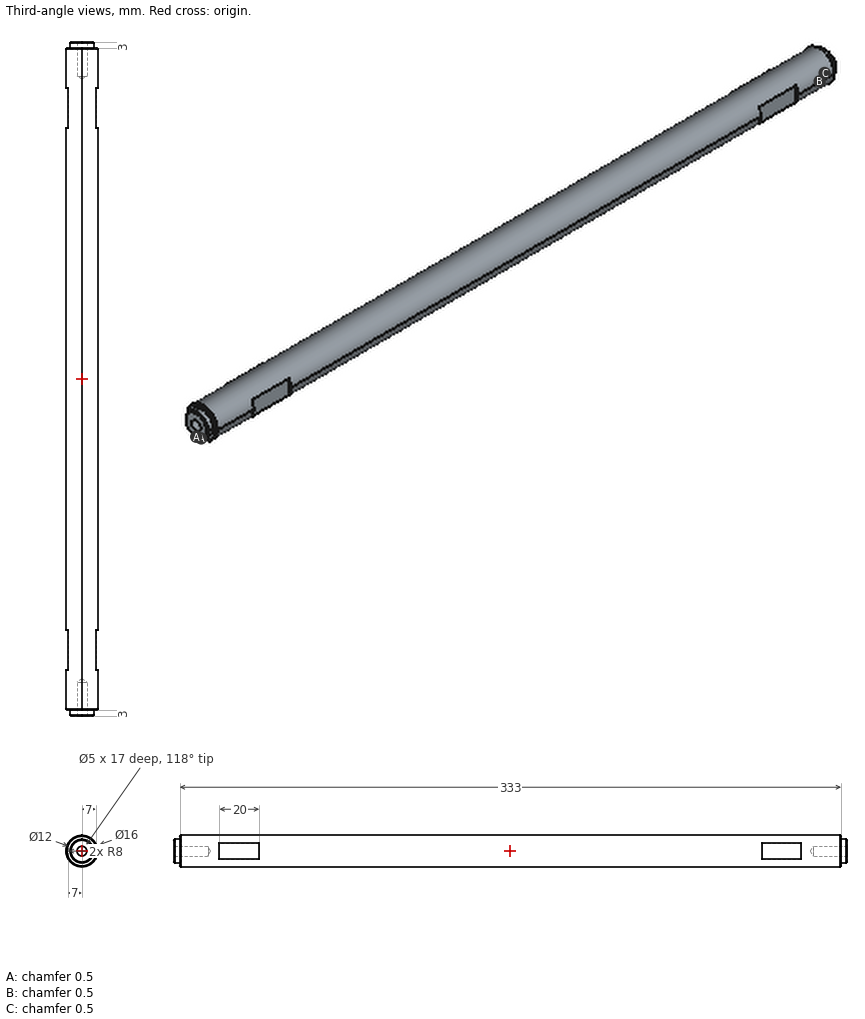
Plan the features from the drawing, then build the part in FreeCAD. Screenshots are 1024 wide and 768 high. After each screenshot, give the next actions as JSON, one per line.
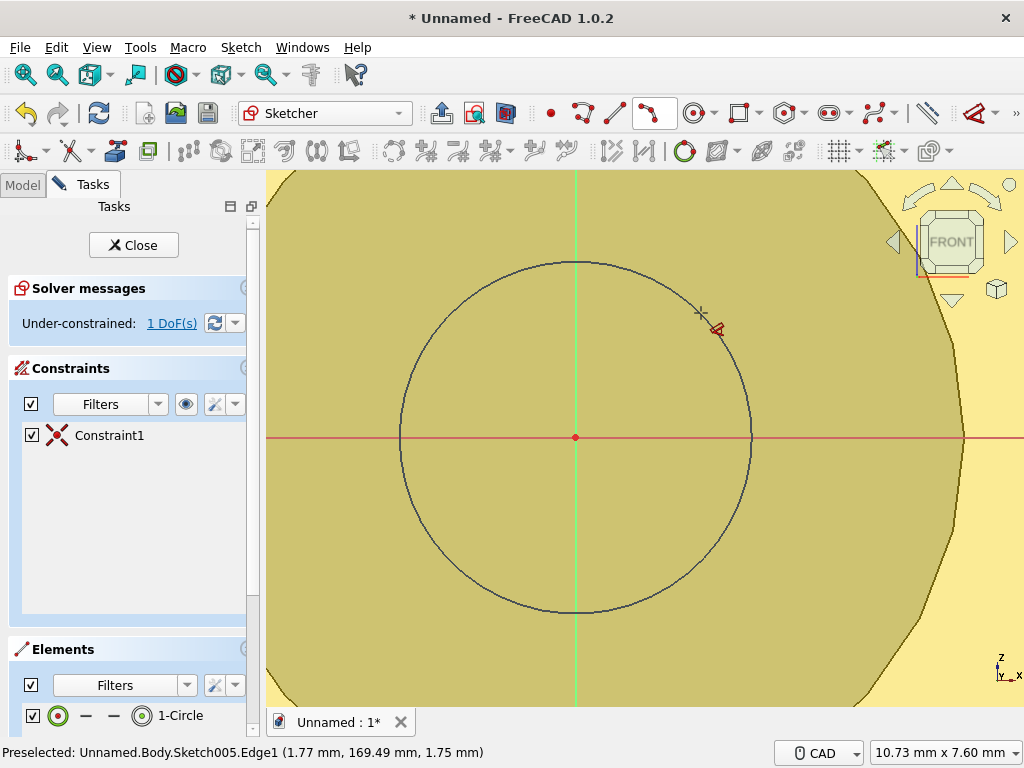
{"action": "left_click", "coordinate": [700, 313]}
{"action": "left_click", "coordinate": [723, 290]}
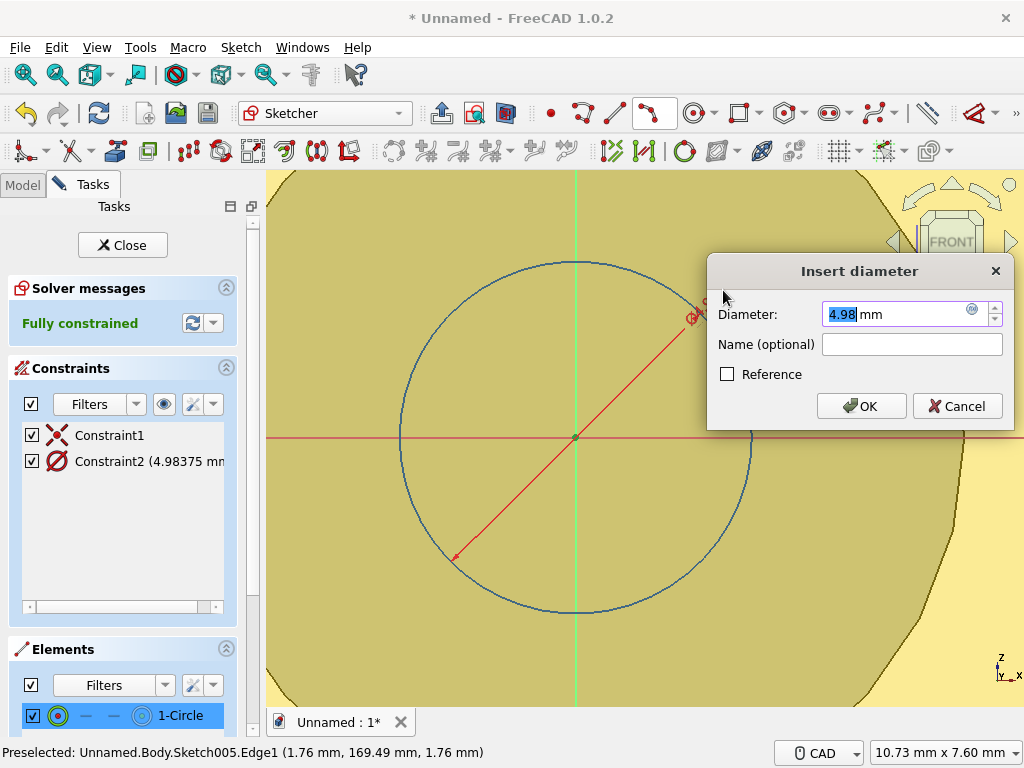
{"action": "type", "text": "5"}
{"action": "key", "text": "Return"}
{"action": "key", "text": "Escape"}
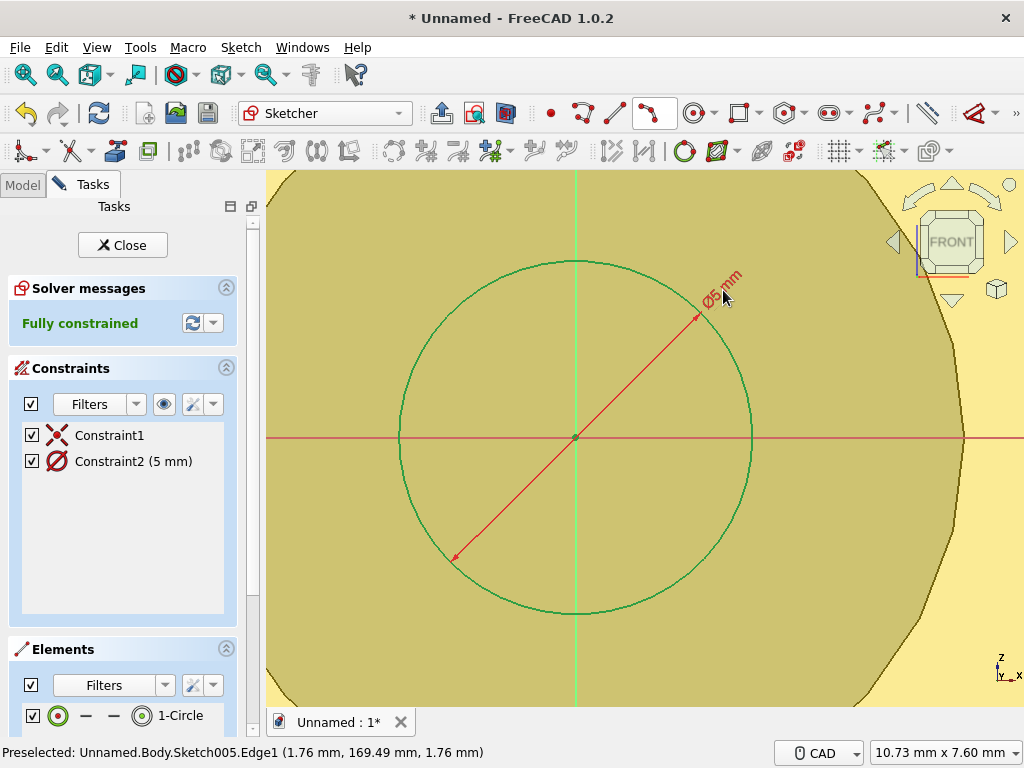
{"action": "left_click", "coordinate": [123, 245]}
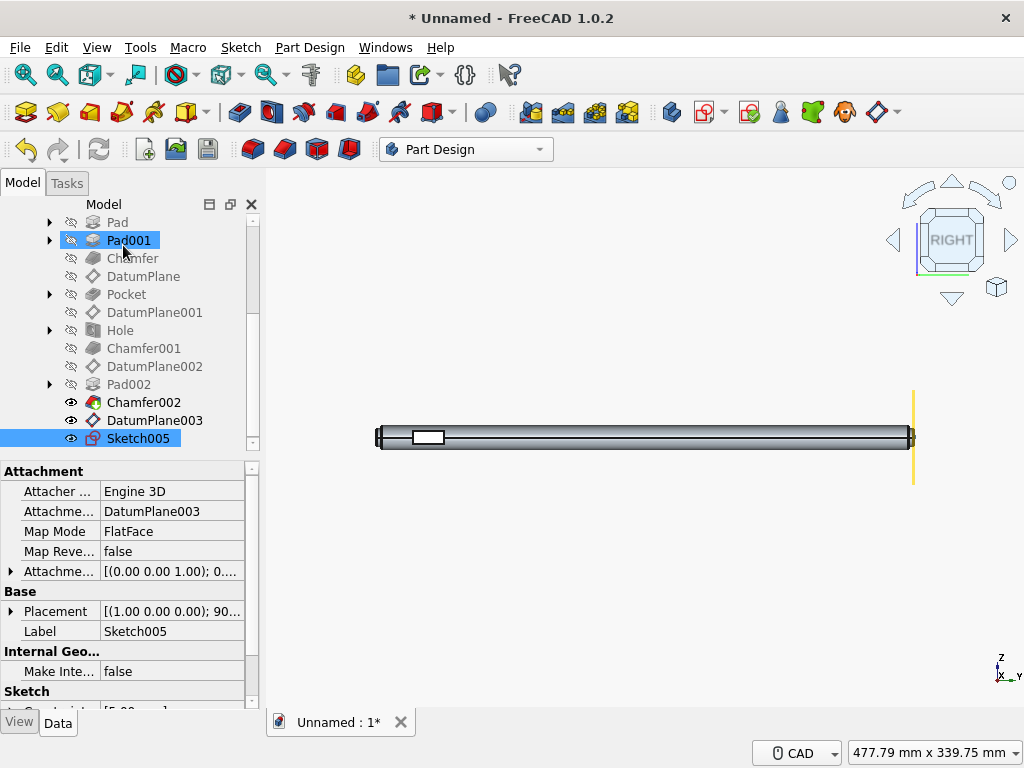
{"action": "left_click", "coordinate": [272, 112]}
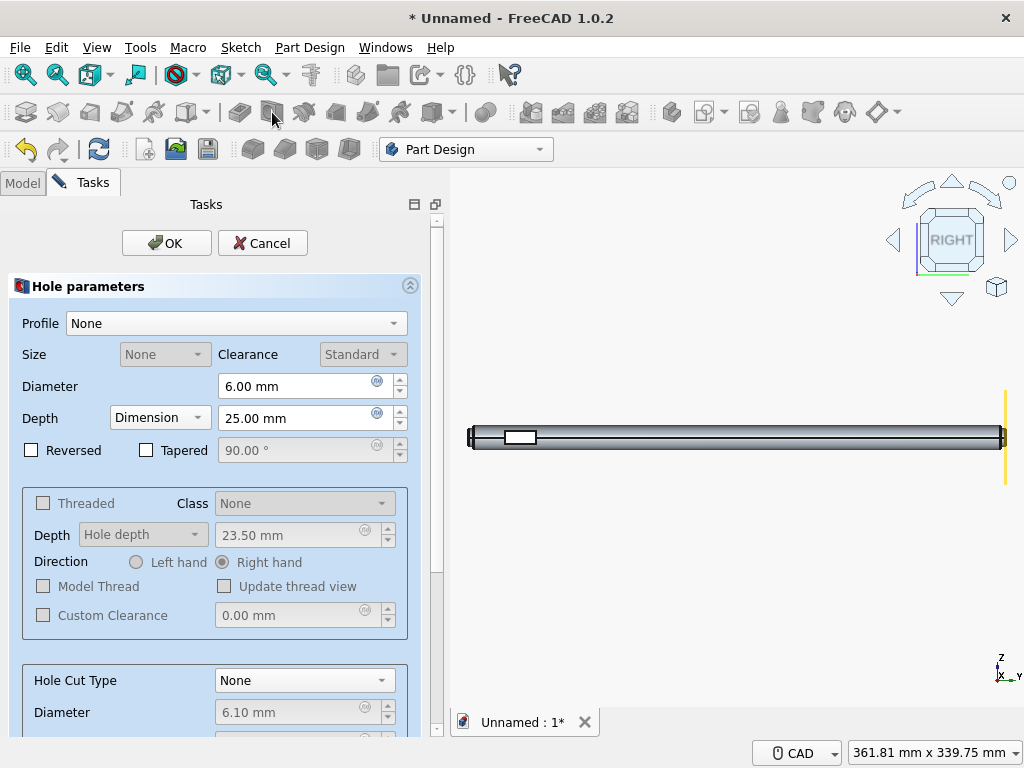
{"action": "triple_click", "coordinate": [305, 386]}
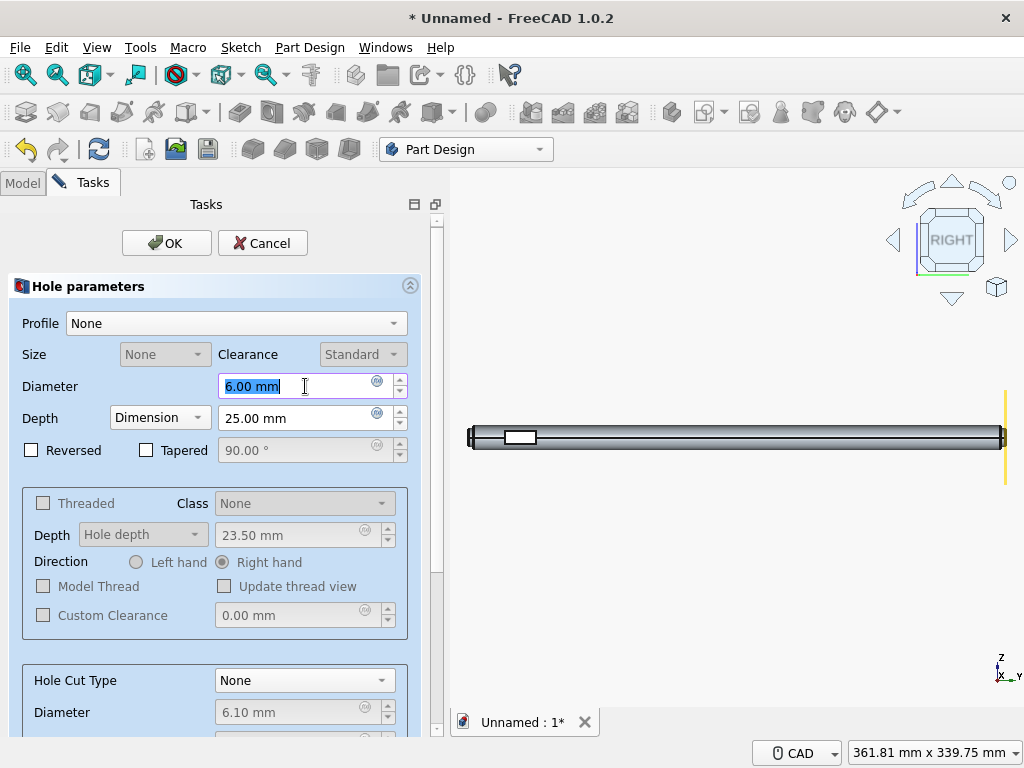
{"action": "type", "text": "5"}
{"action": "key", "text": "Tab"}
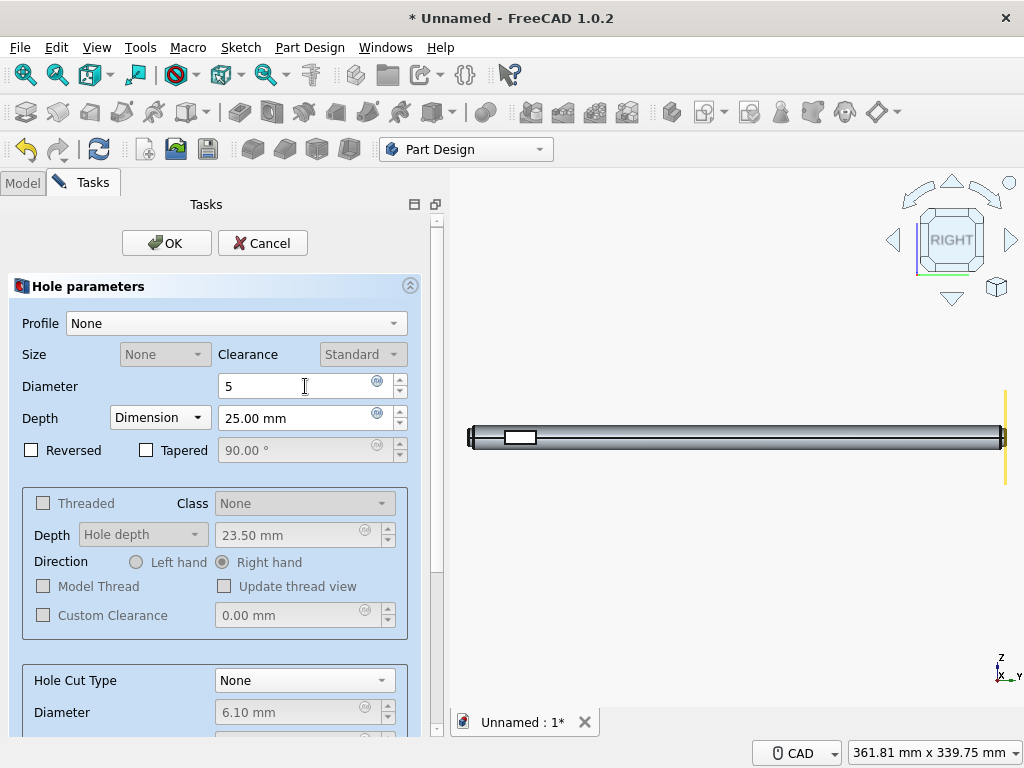
{"action": "triple_click", "coordinate": [305, 418]}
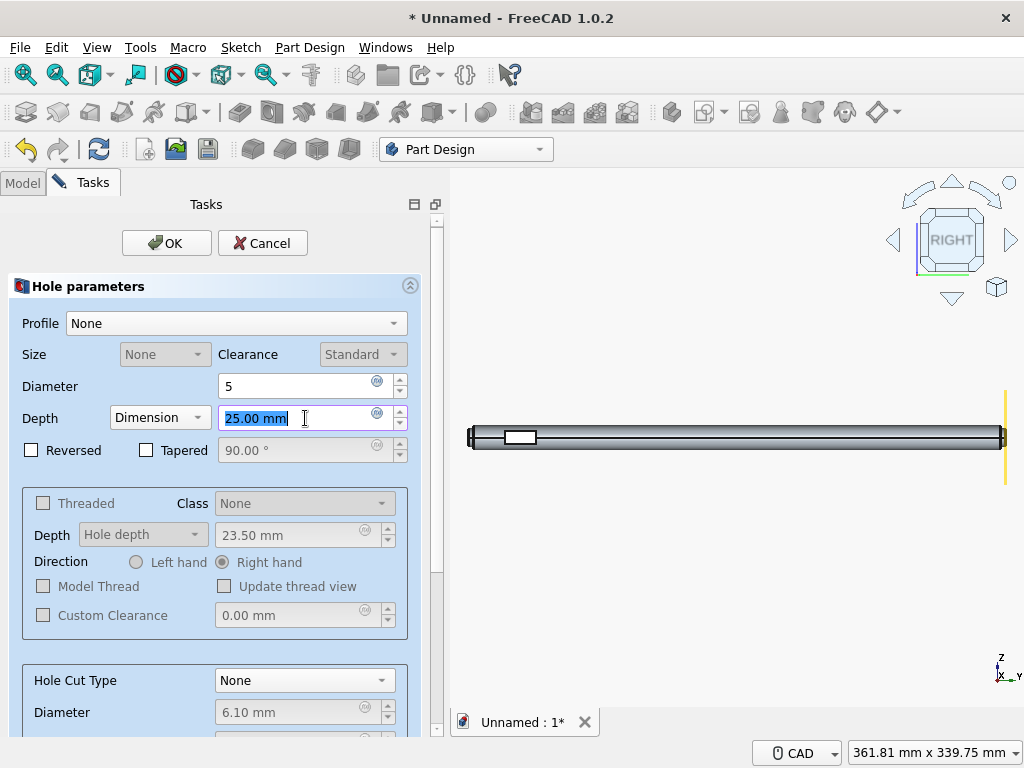
{"action": "type", "text": "17"}
{"action": "key", "text": "Tab"}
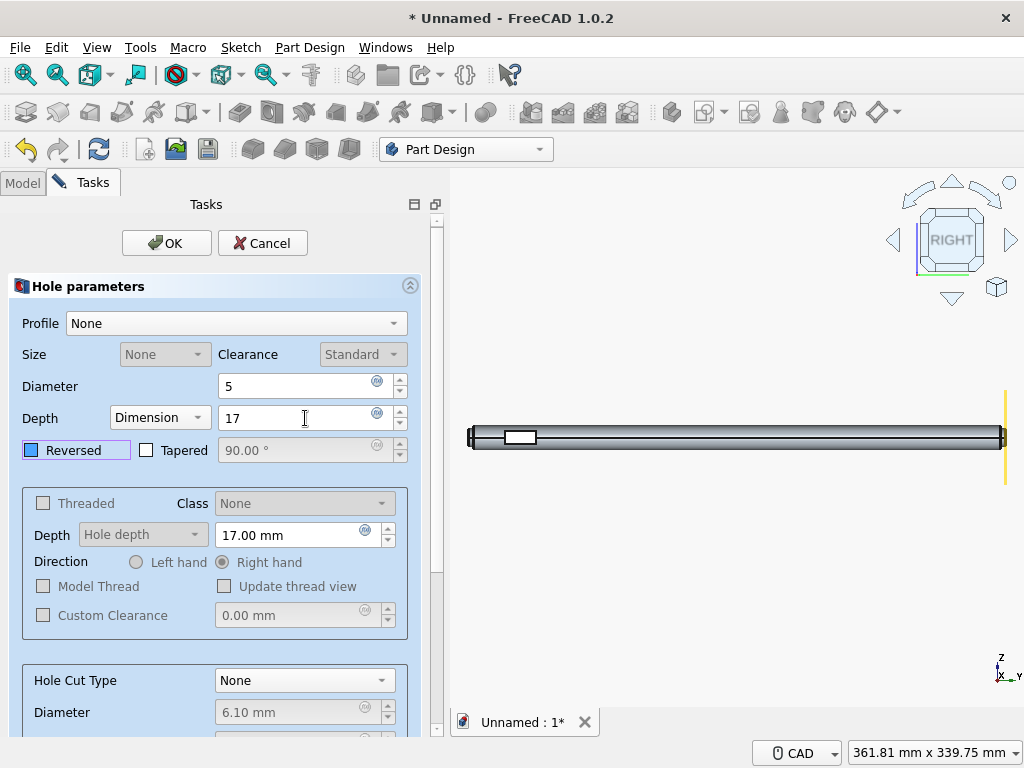
{"action": "left_click", "coordinate": [30, 450]}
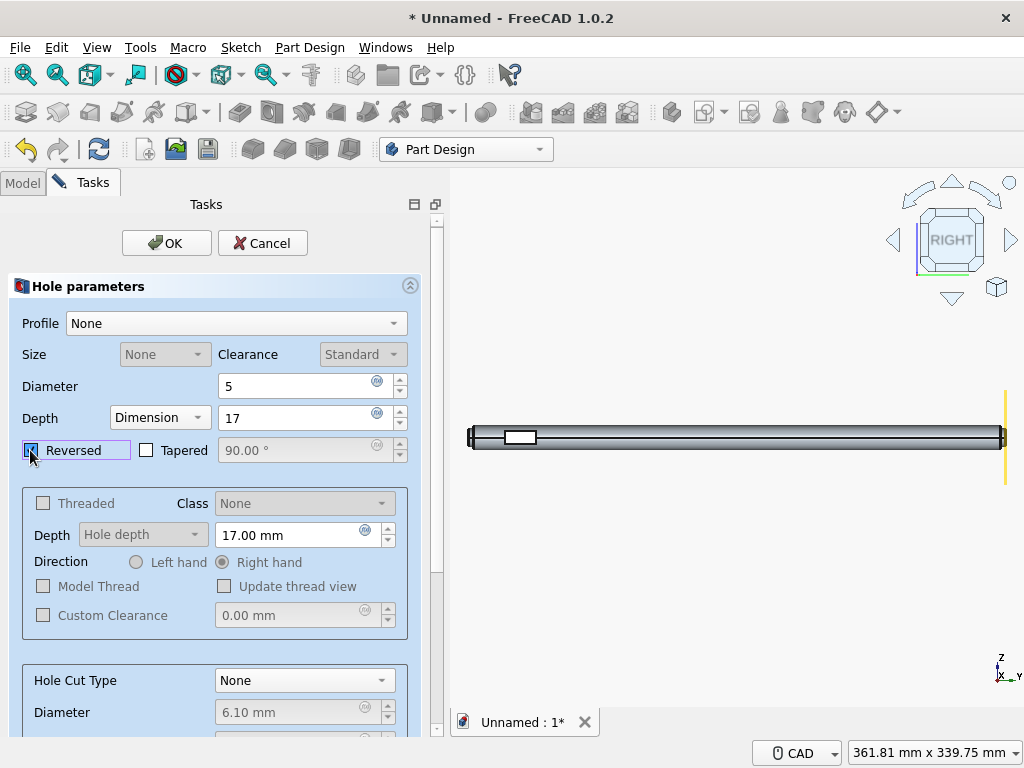
{"action": "left_click", "coordinate": [167, 243]}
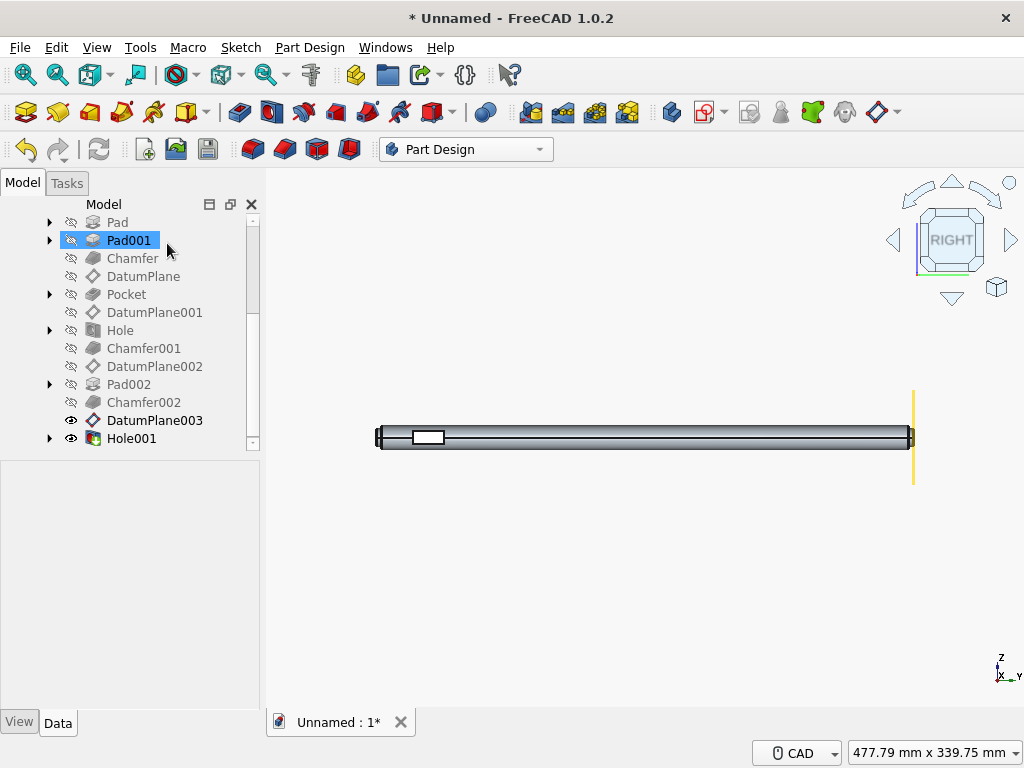
{"action": "left_click", "coordinate": [116, 420]}
{"action": "key", "text": "space"}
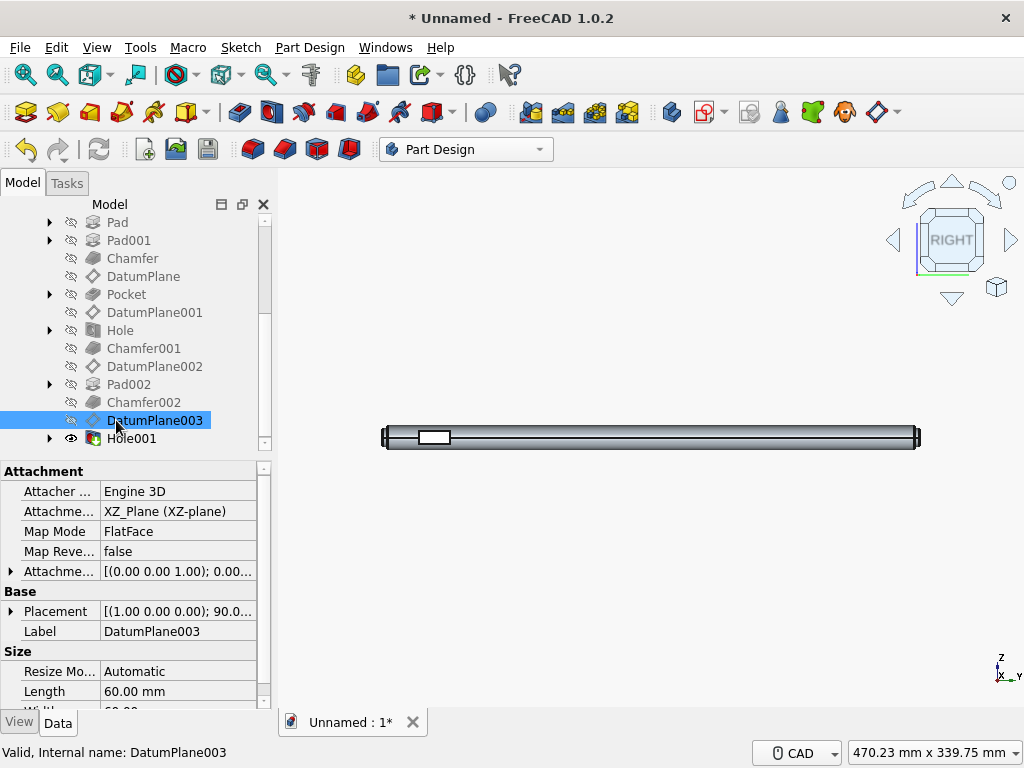
{"action": "left_click", "coordinate": [116, 294]}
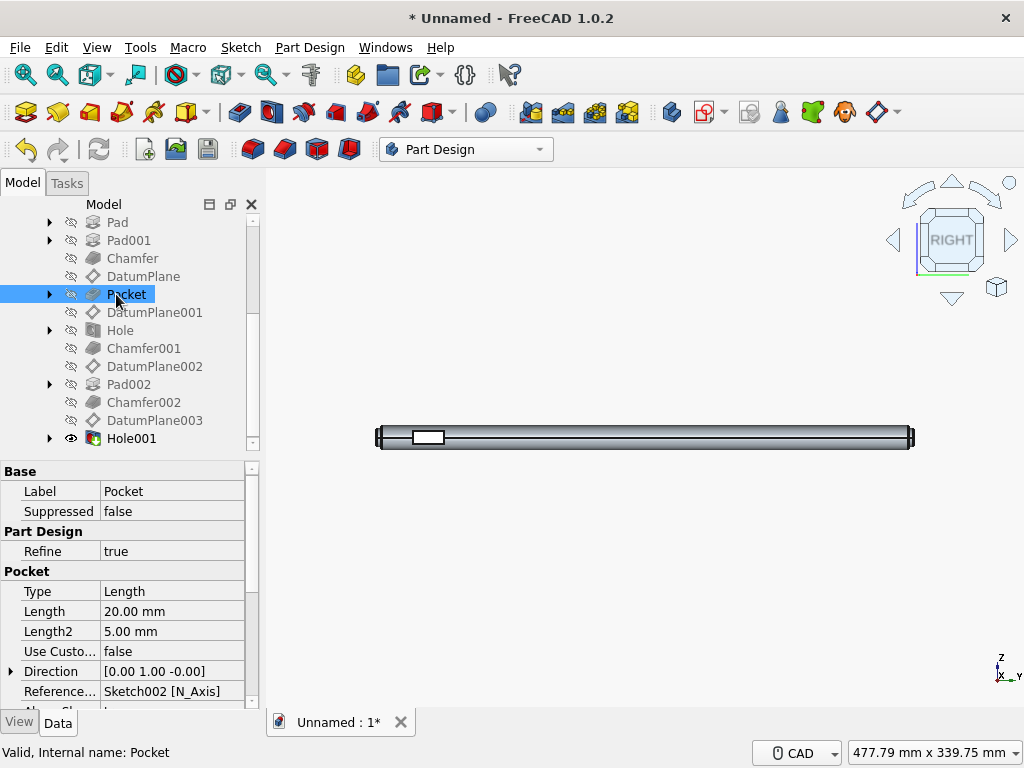
{"action": "left_click", "coordinate": [532, 112]}